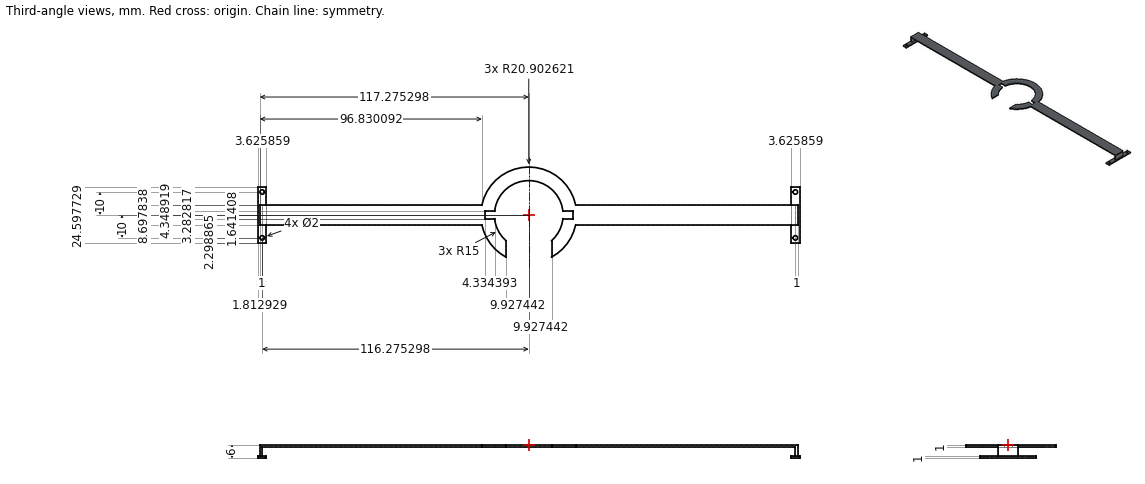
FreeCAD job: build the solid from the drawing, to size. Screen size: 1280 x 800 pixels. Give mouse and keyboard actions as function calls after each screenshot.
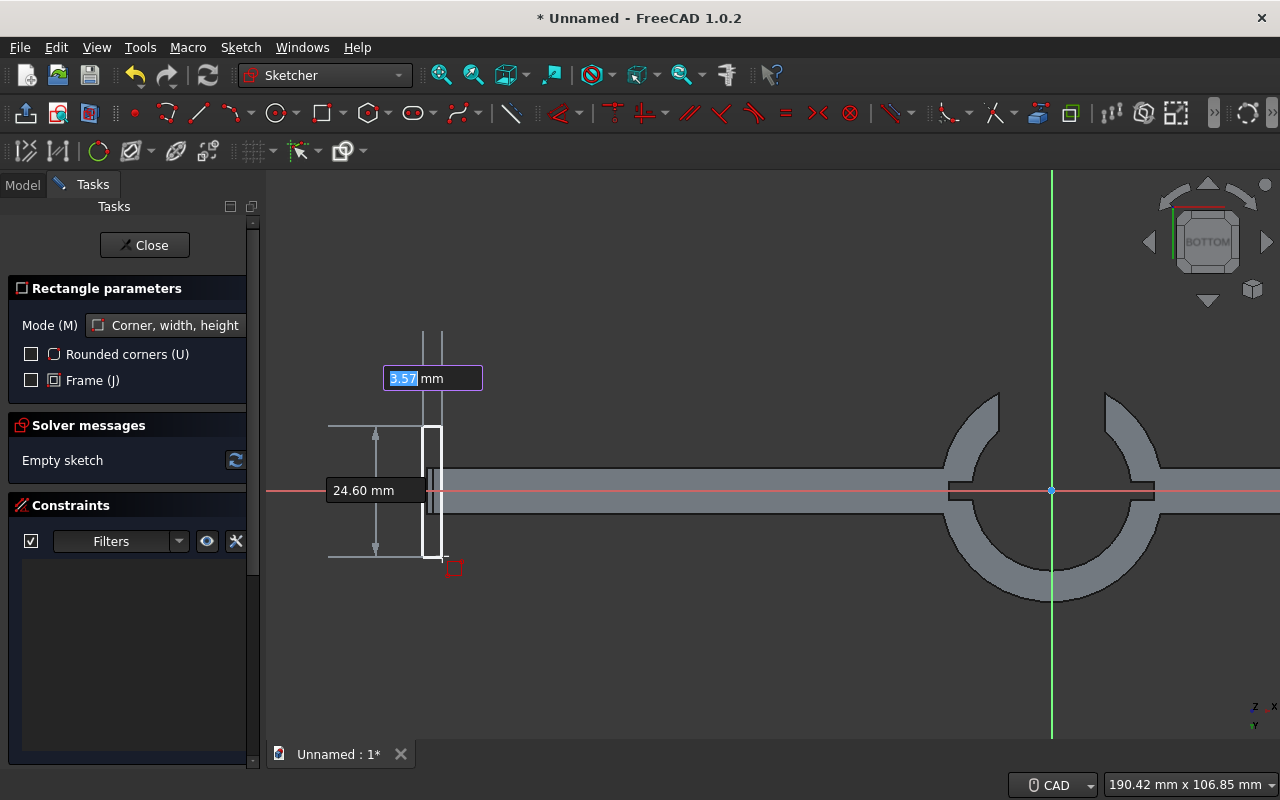
text(3.625859)
key(Tab)
text(24.597729)
key(Return)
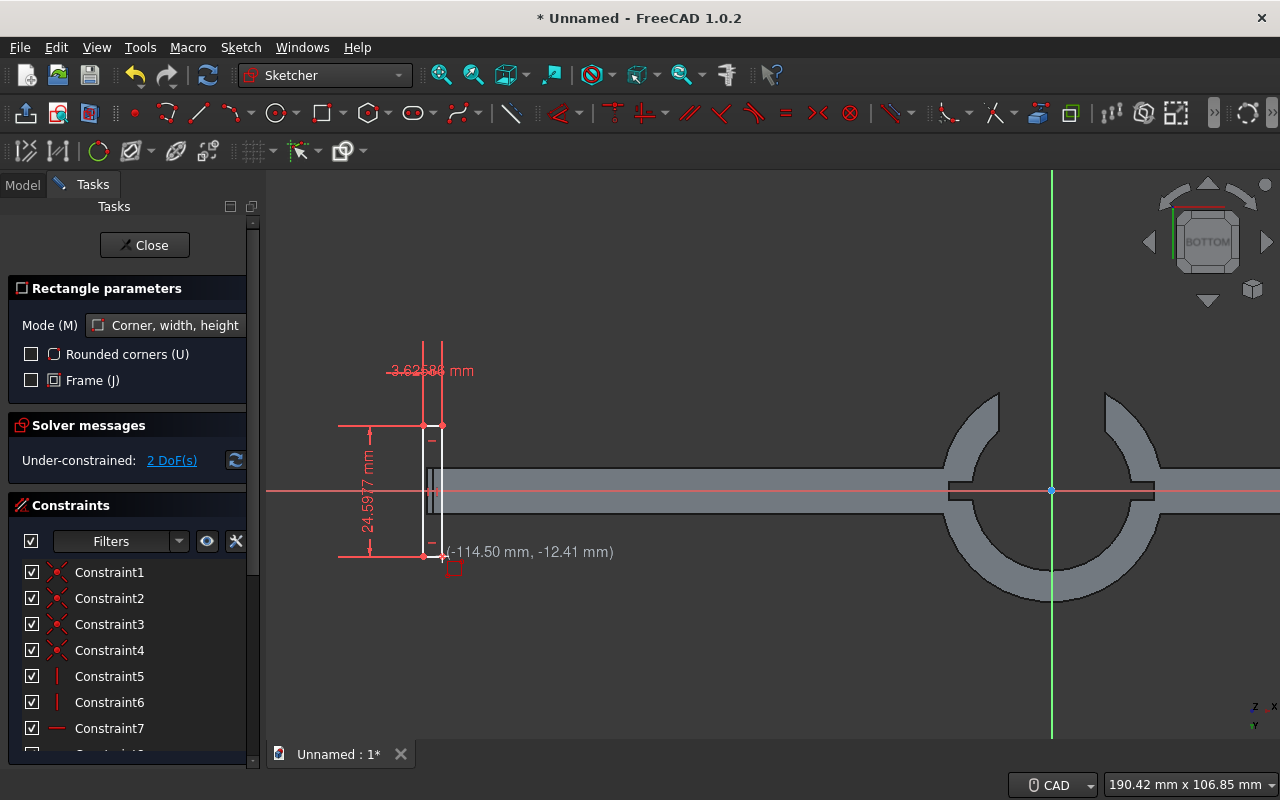
scroll(421, 425, down, 4)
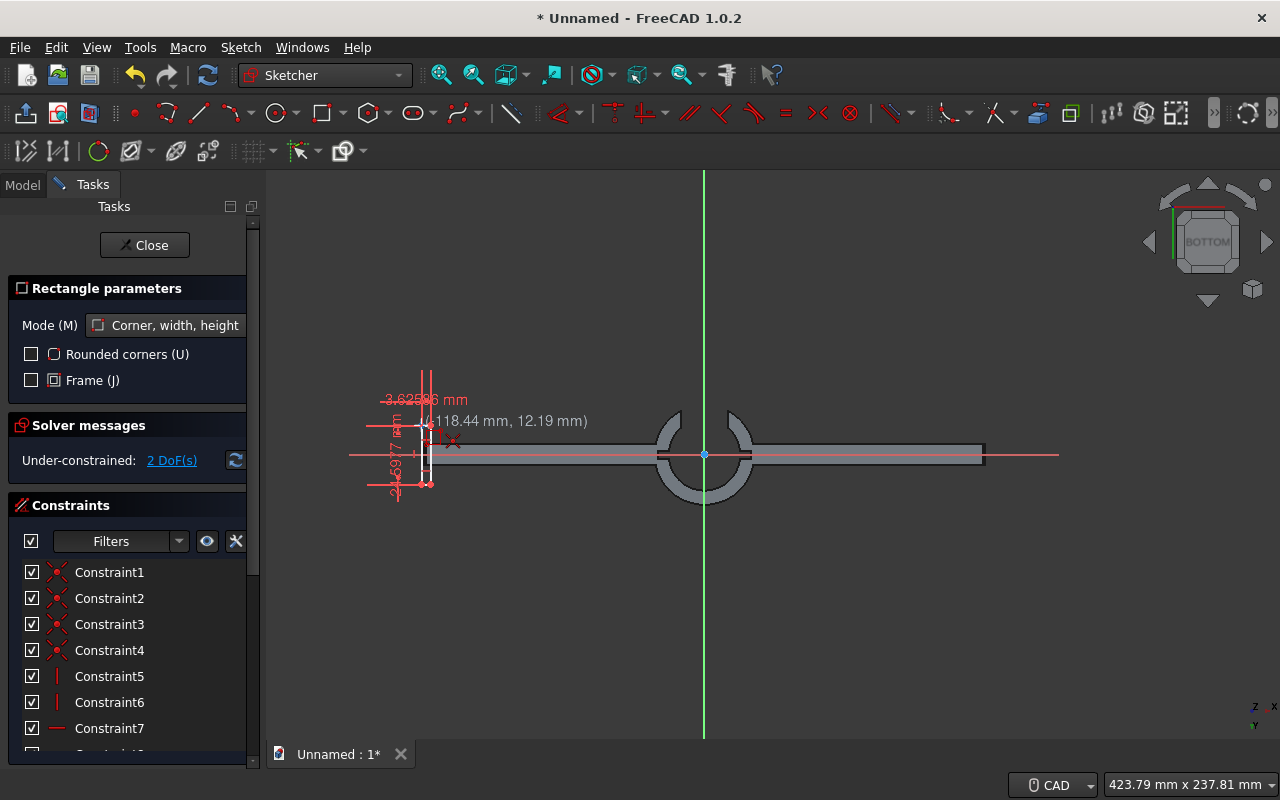
scroll(978, 425, up, 4)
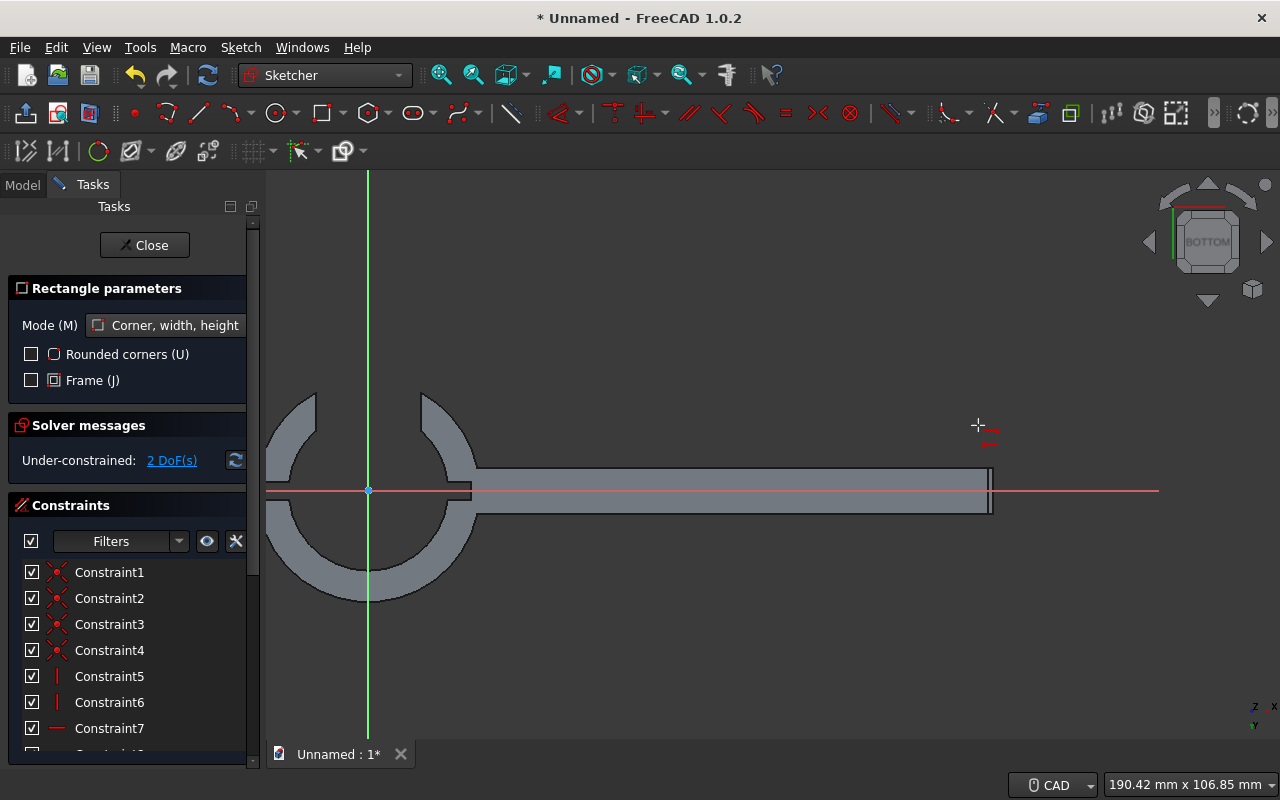
click(978, 425)
move(997, 556)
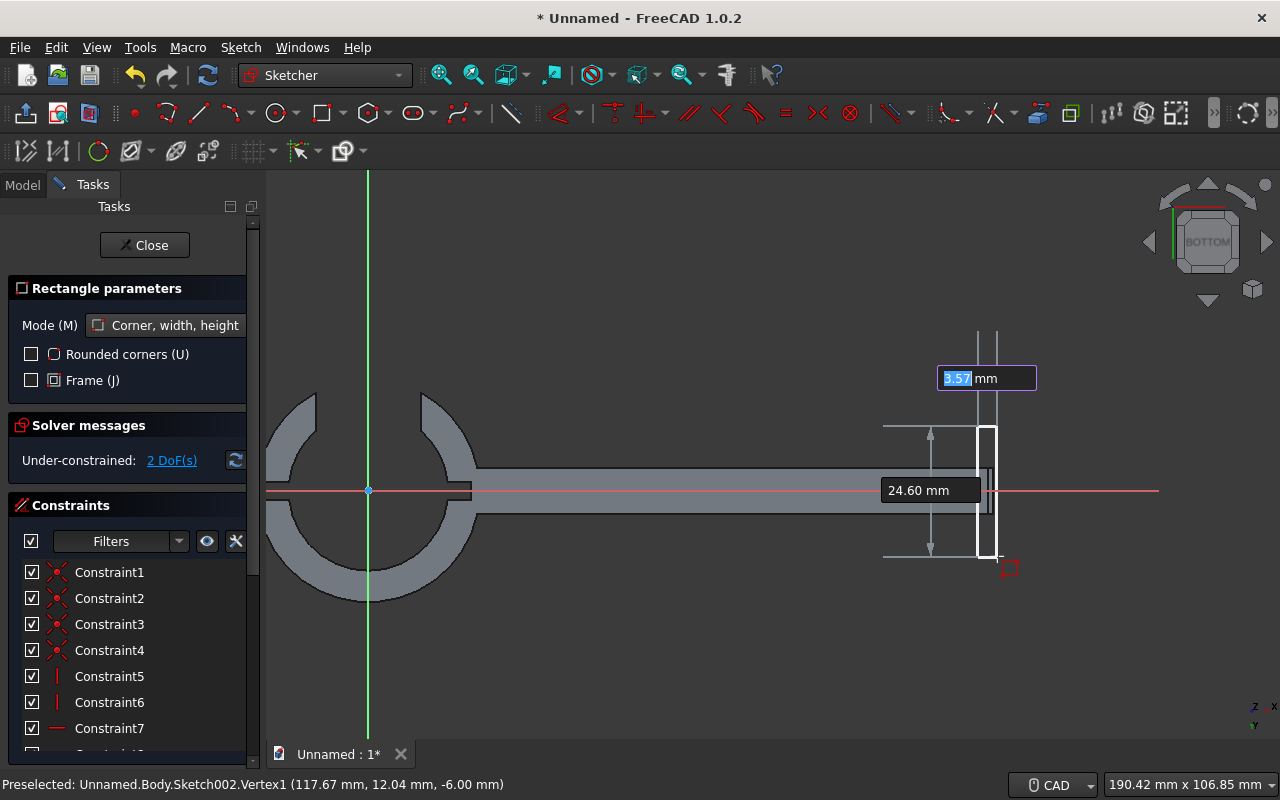
text(3.625859)
key(Tab)
text(24.597729)
key(Return)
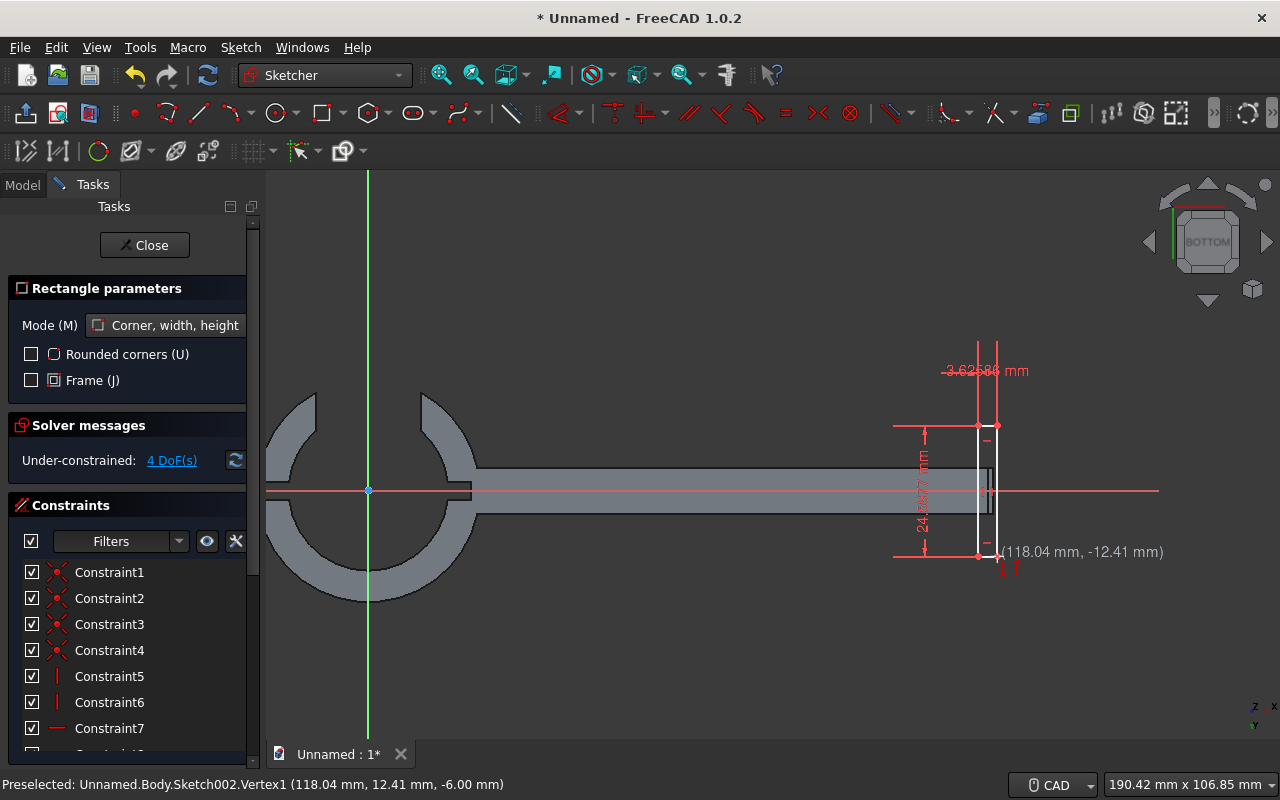
click(276, 114)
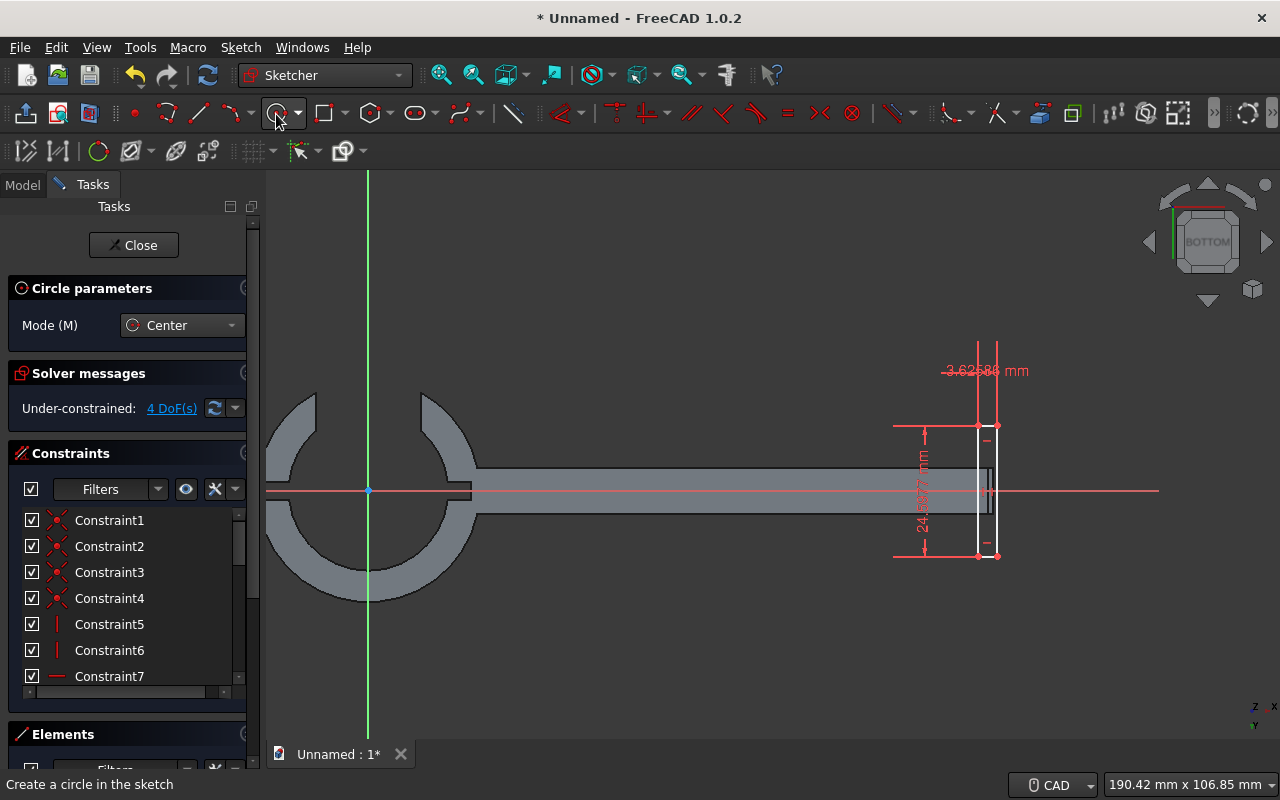
scroll(979, 425, down, 4)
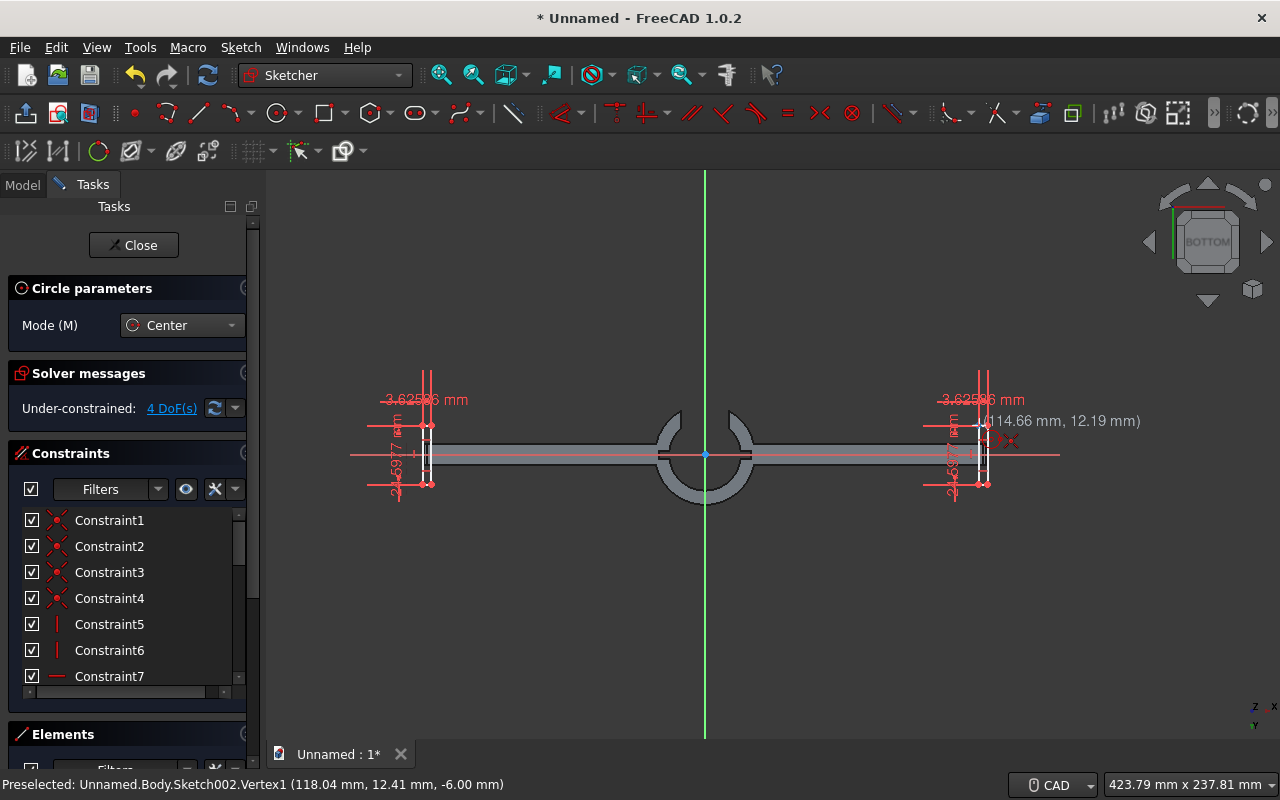
scroll(427, 431, up, 12)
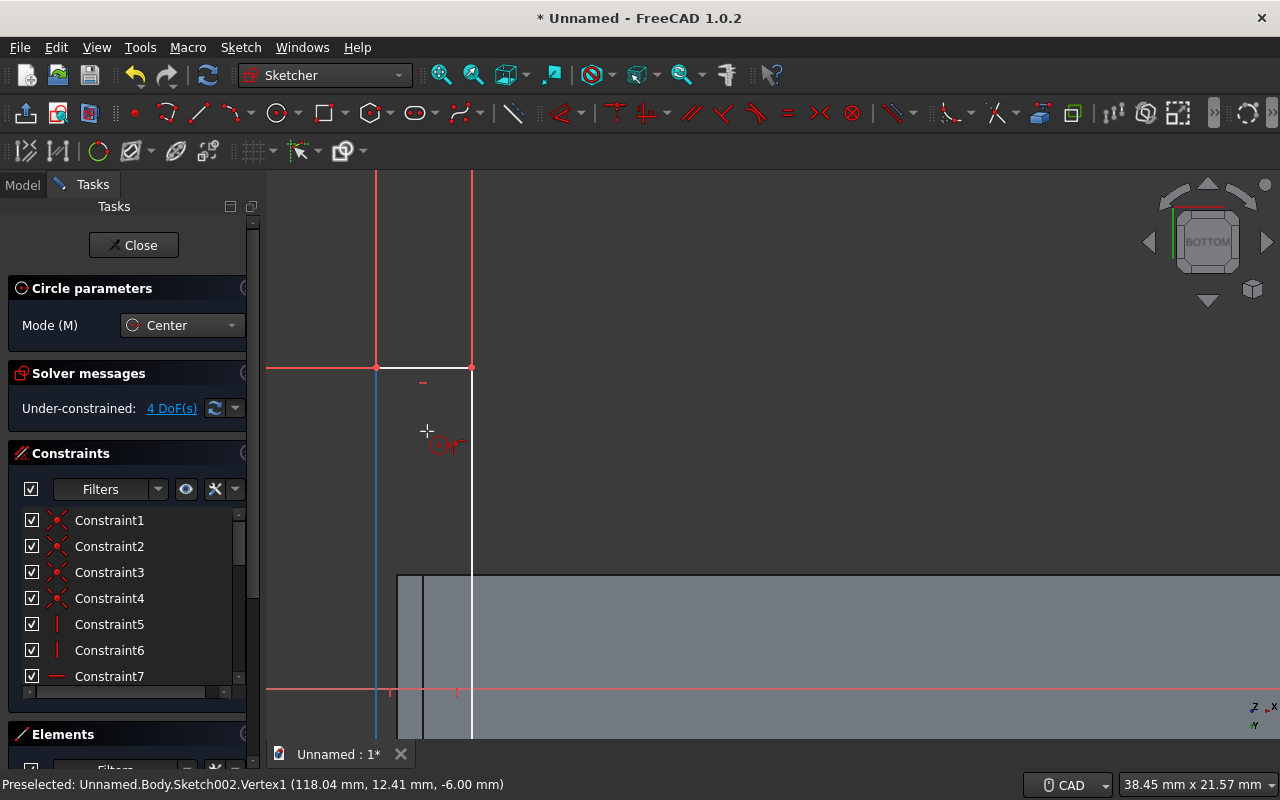
scroll(427, 431, down, 12)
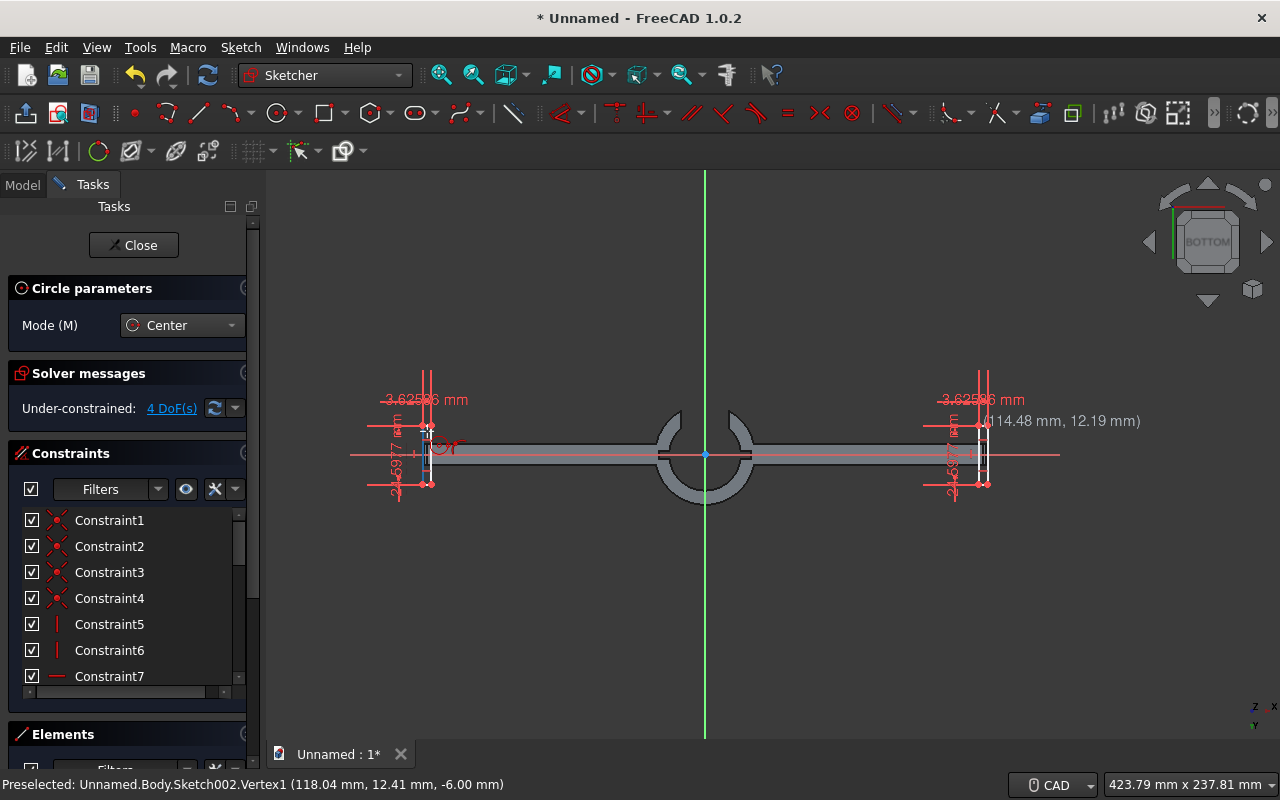
scroll(427, 431, up, 7)